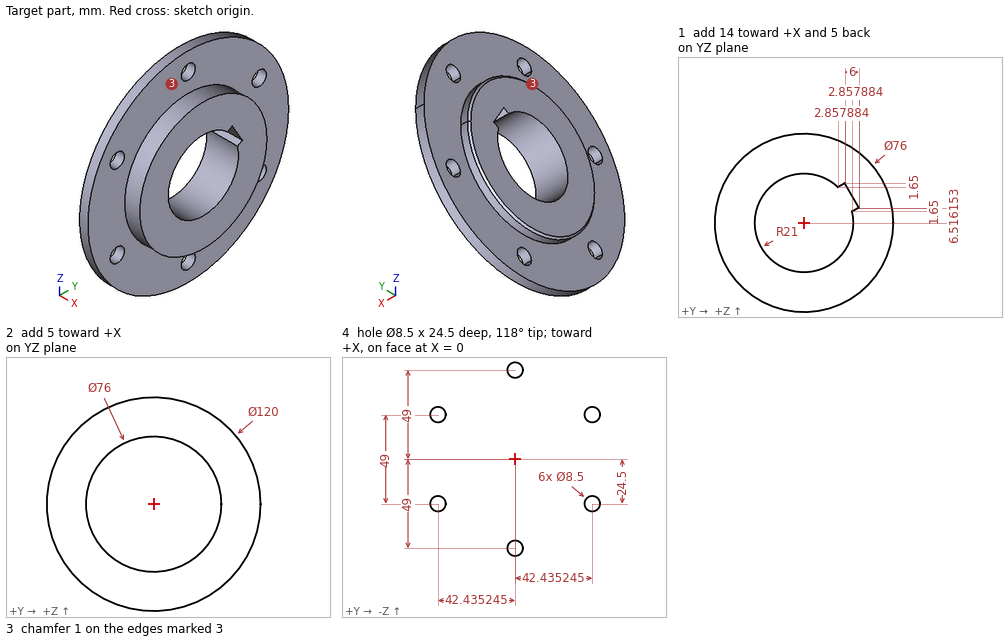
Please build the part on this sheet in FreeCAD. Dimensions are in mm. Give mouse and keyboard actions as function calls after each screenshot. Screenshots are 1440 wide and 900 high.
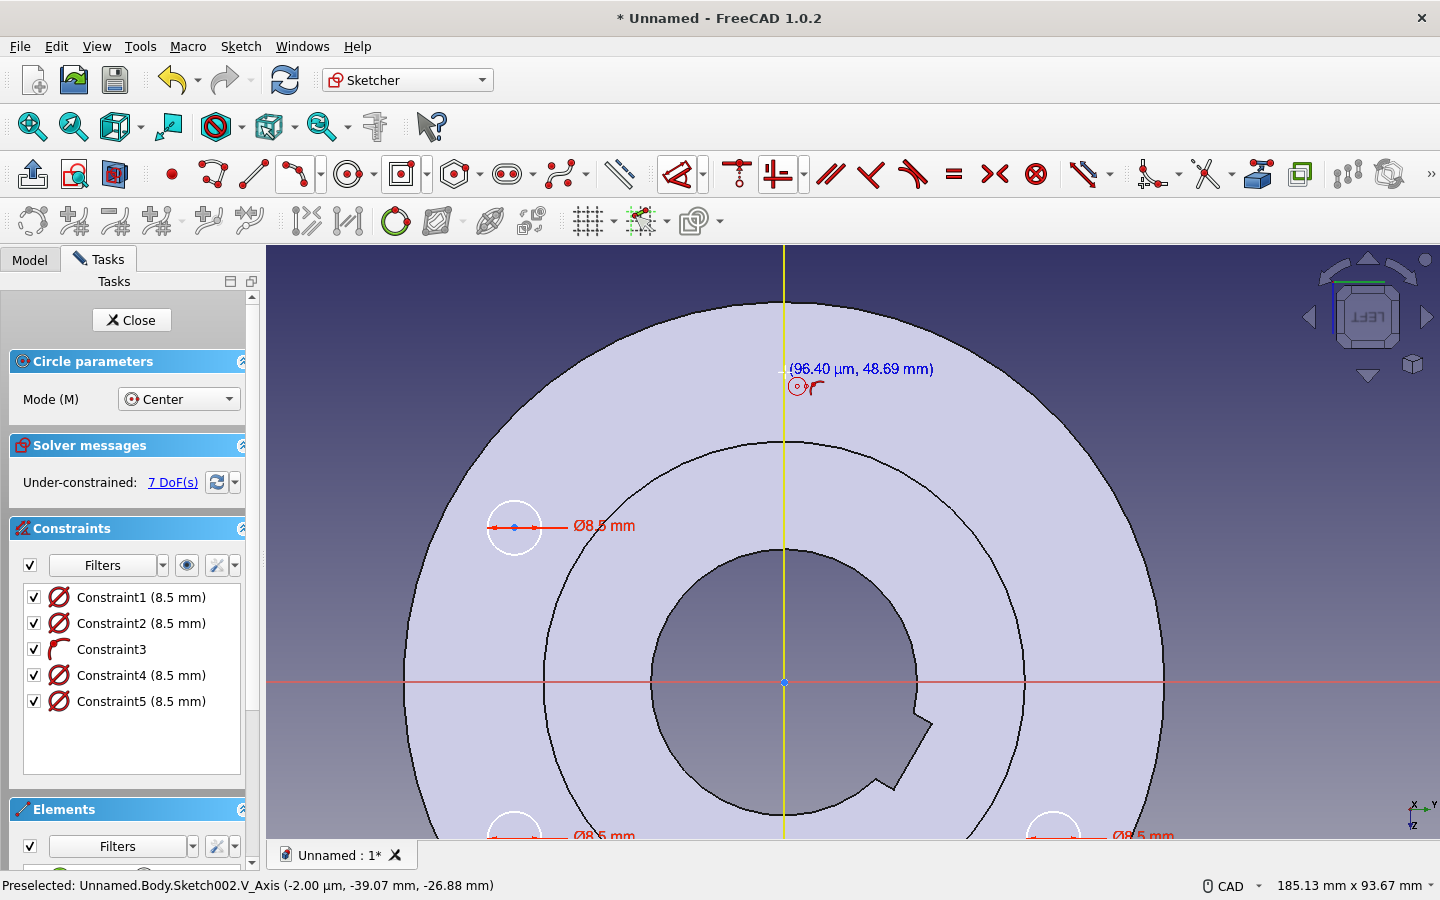
click(784, 372)
move(803, 353)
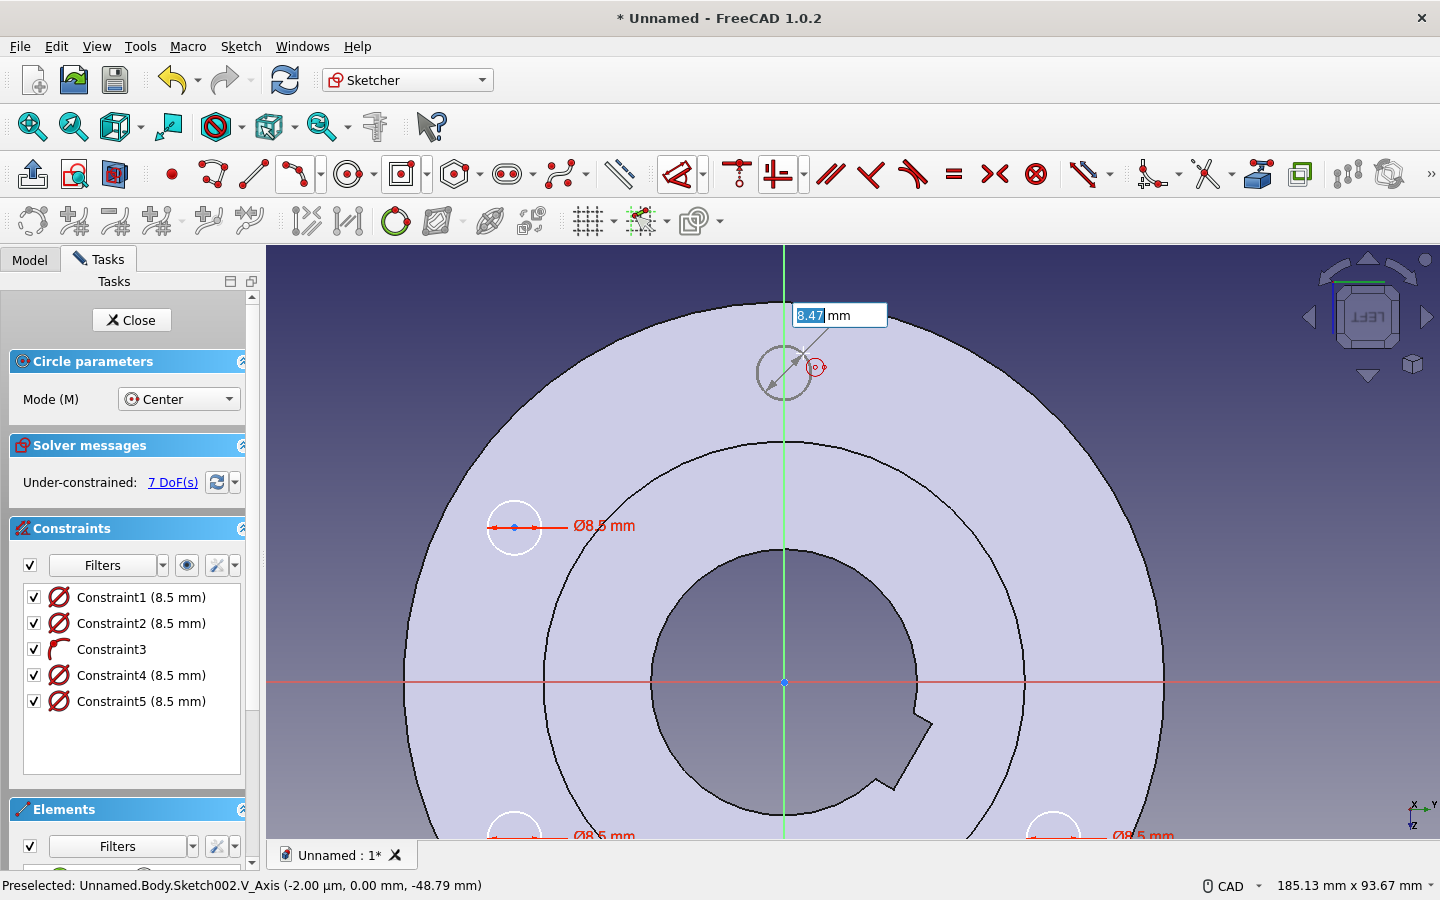
text(8.5)
key(Return)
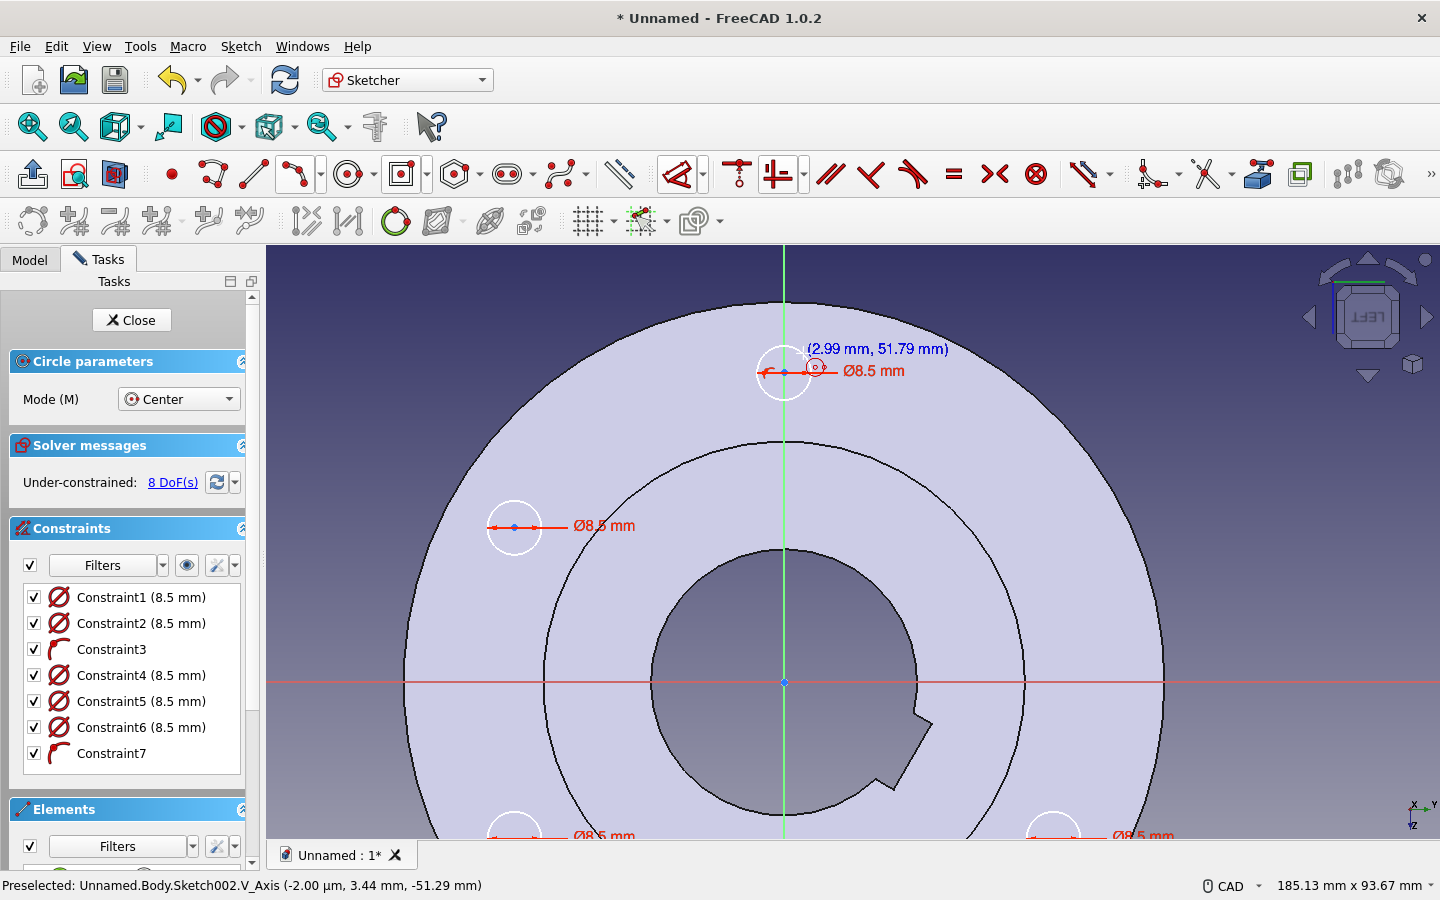
click(1053, 527)
move(1072, 508)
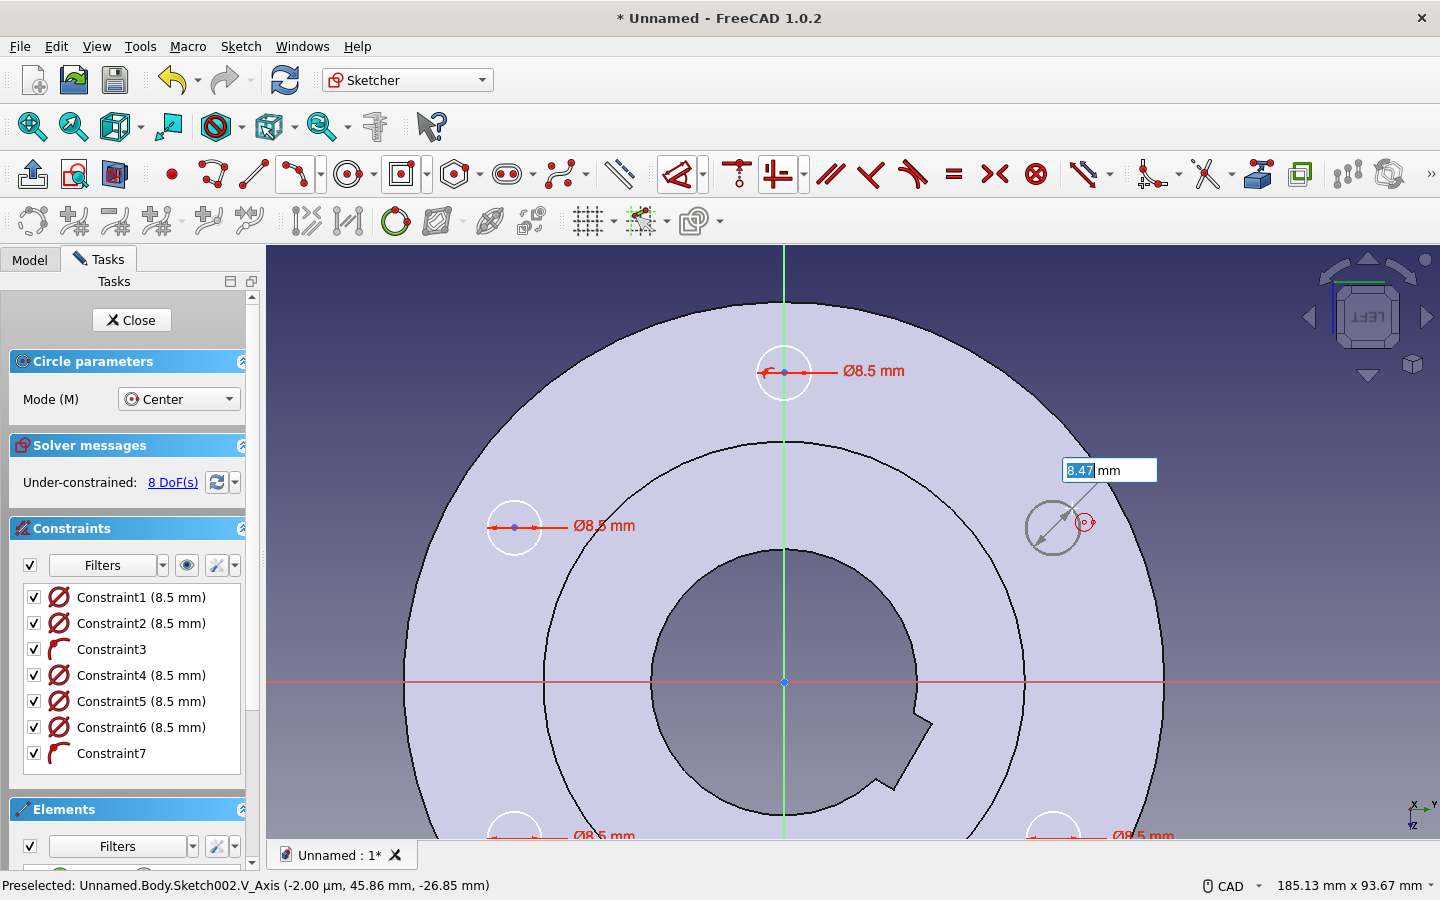
text(8.5)
key(Return)
key(Escape)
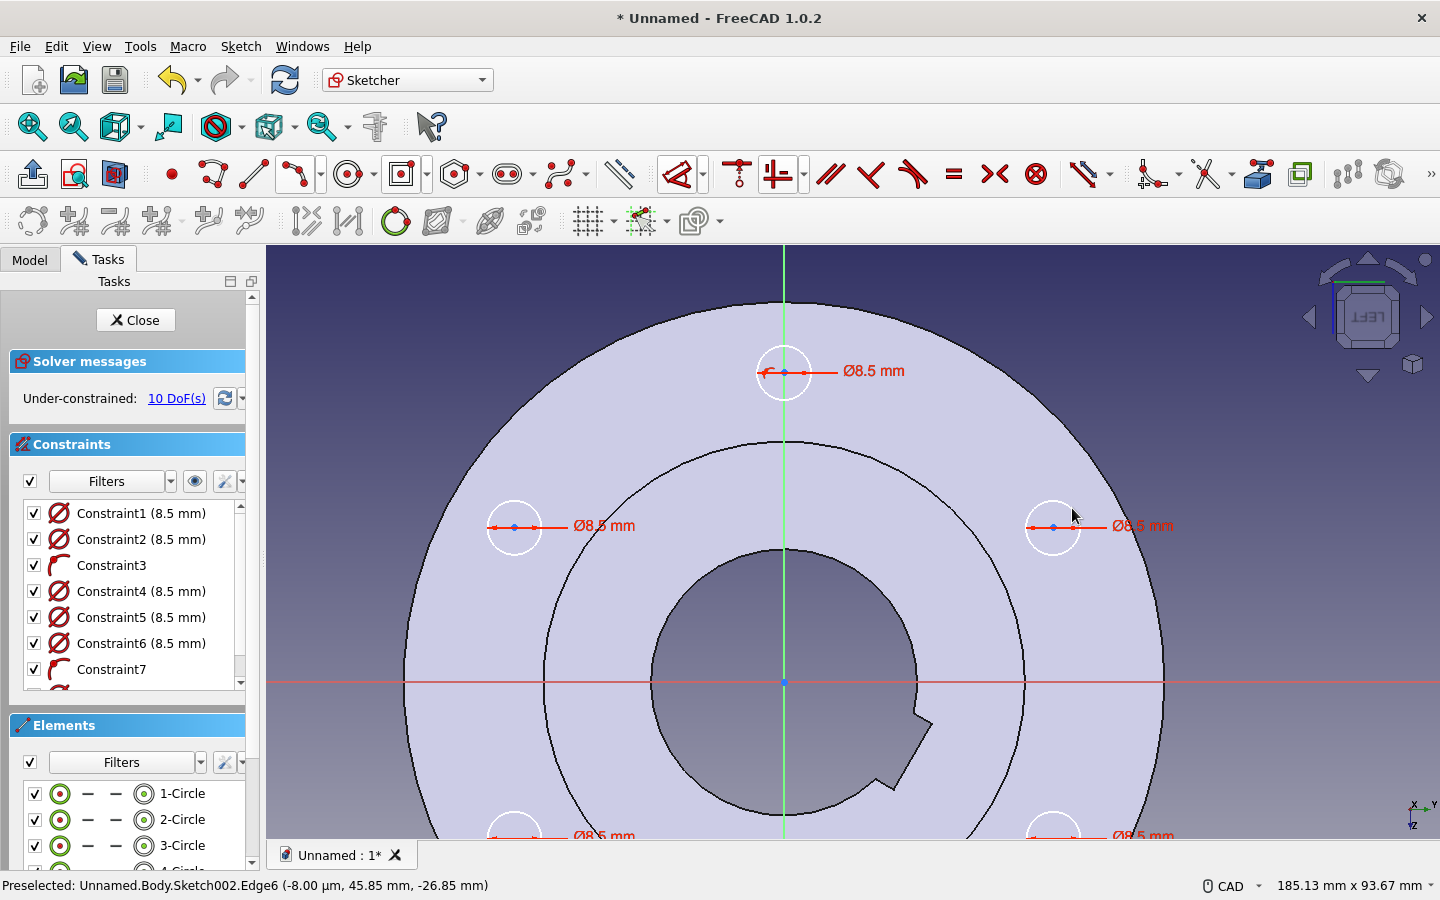
scroll(785, 371, down, 3)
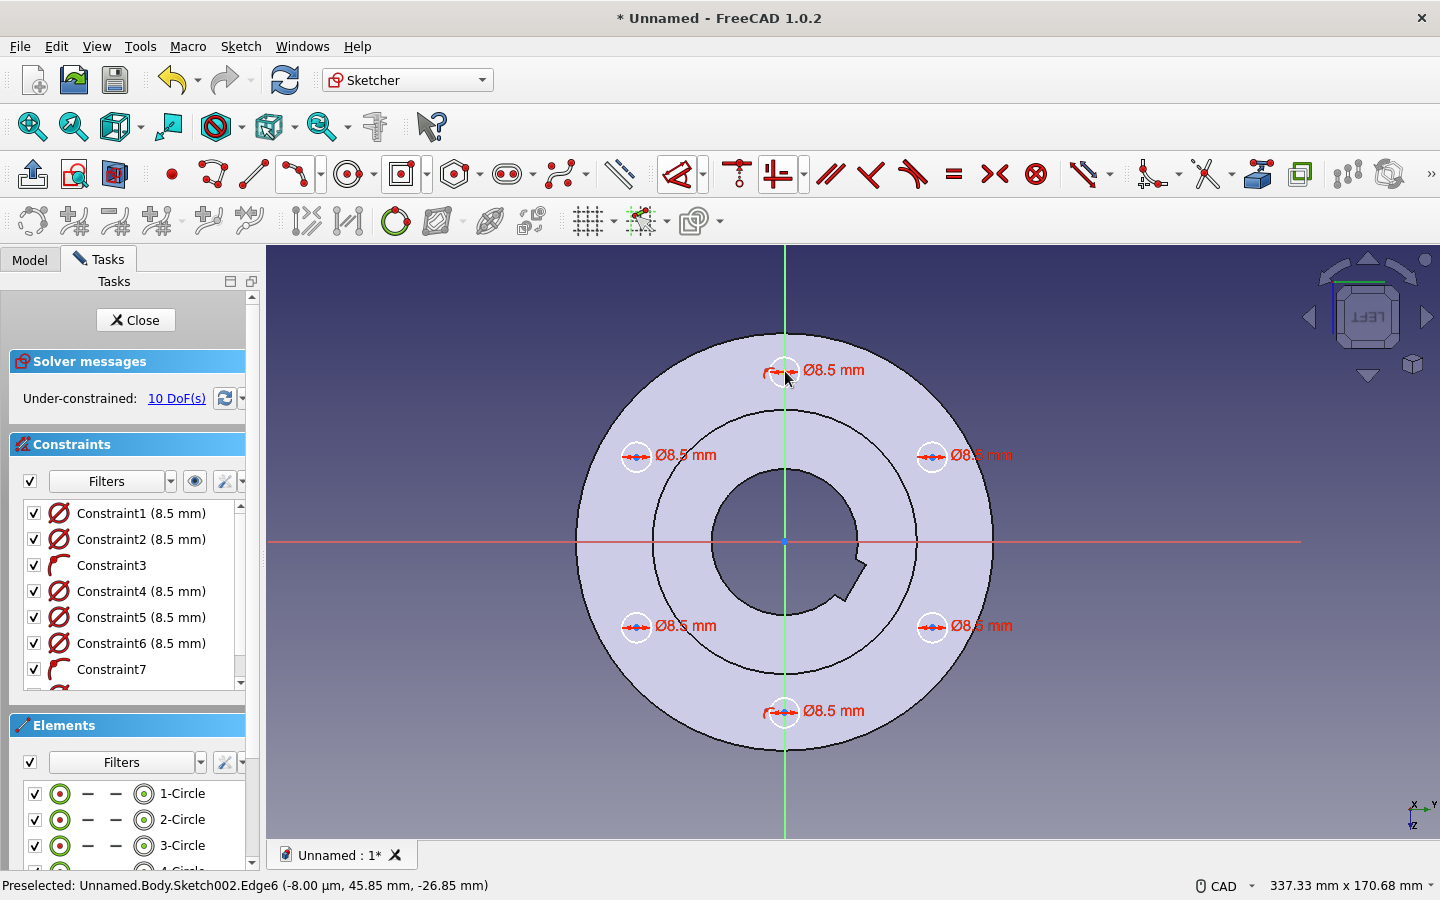
click(933, 628)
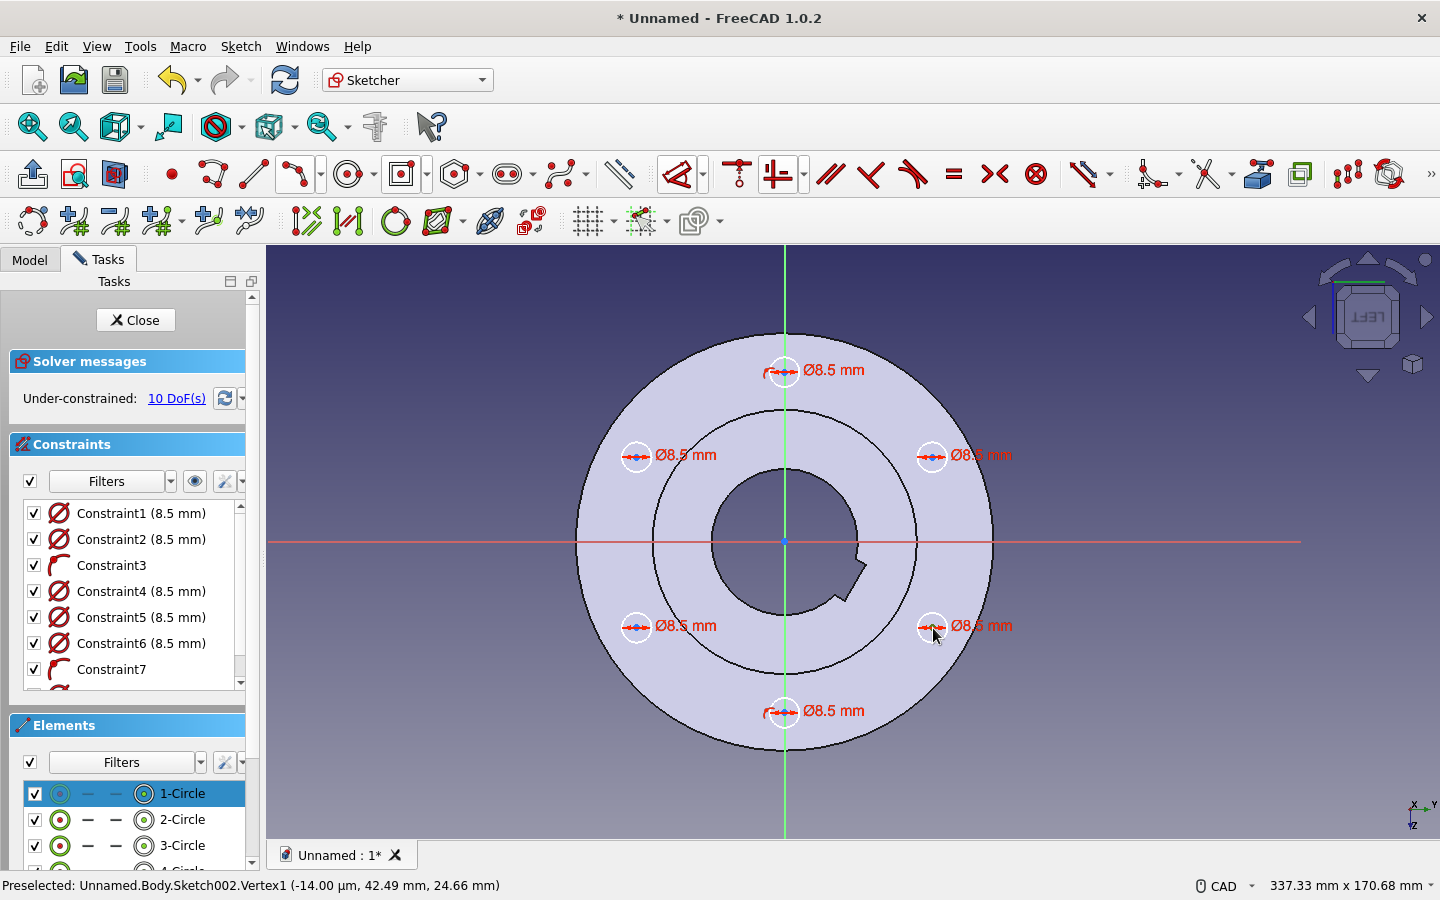
click(637, 628)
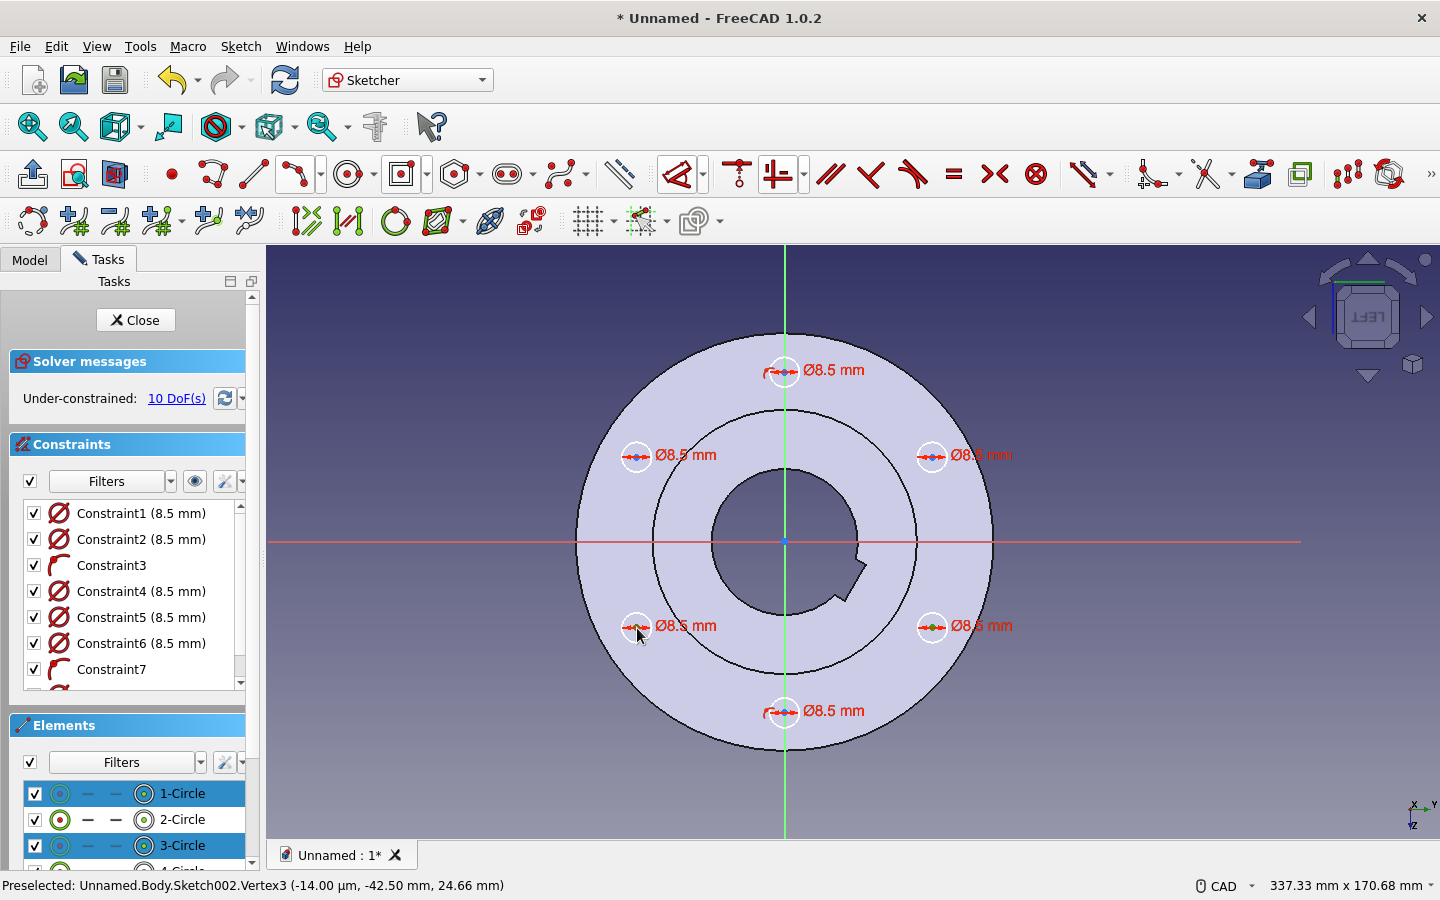
click(804, 174)